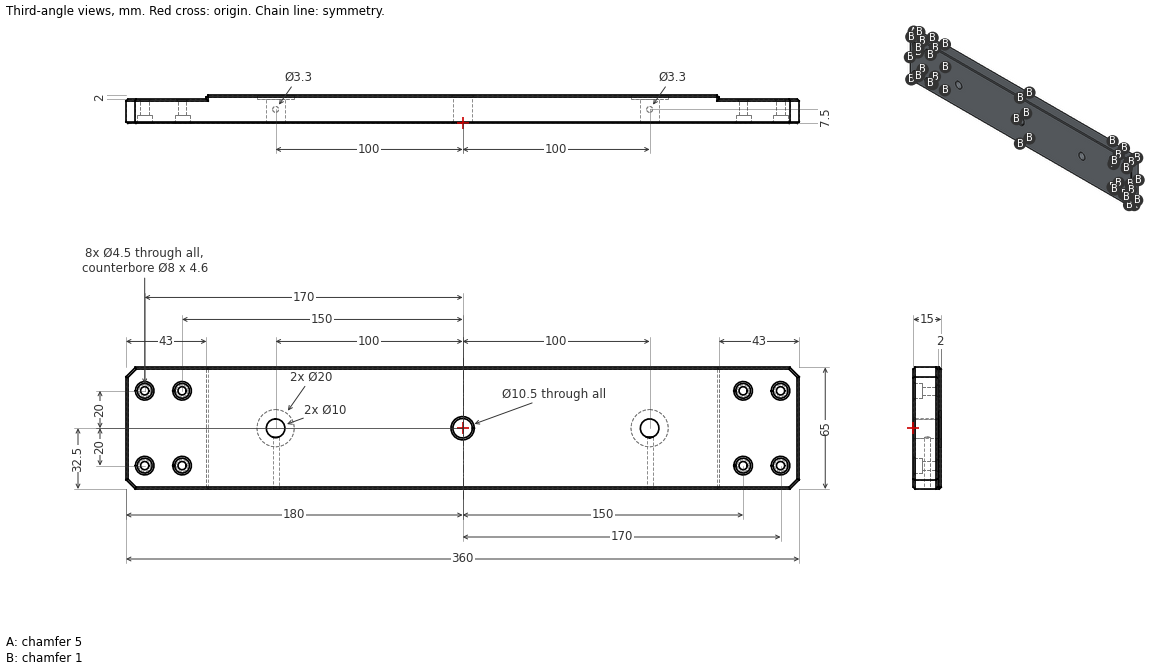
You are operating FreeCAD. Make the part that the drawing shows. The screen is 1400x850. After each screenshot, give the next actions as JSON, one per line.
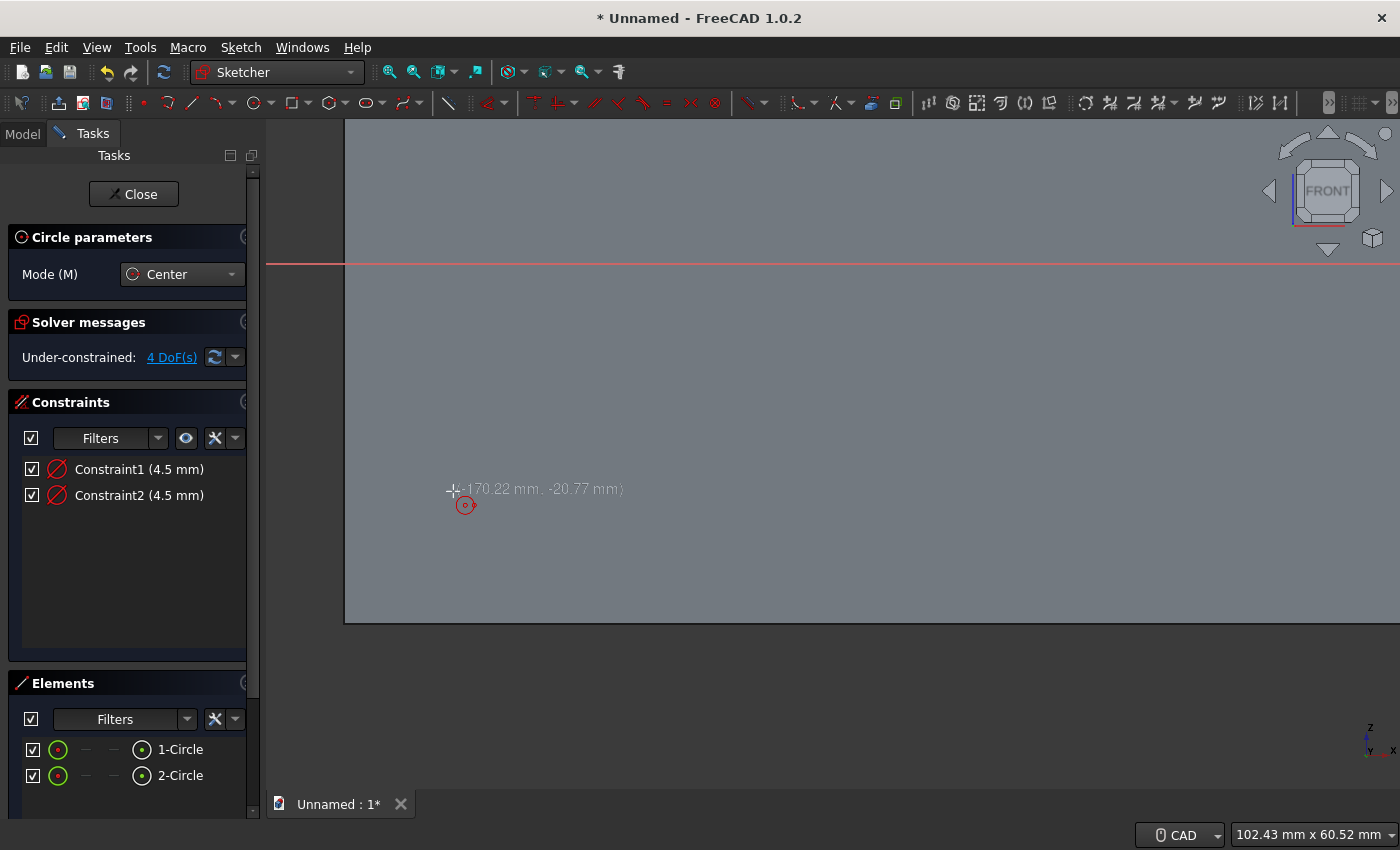
{"action": "scroll", "coordinate": [453, 492], "scroll_direction": "down", "scroll_amount": 9}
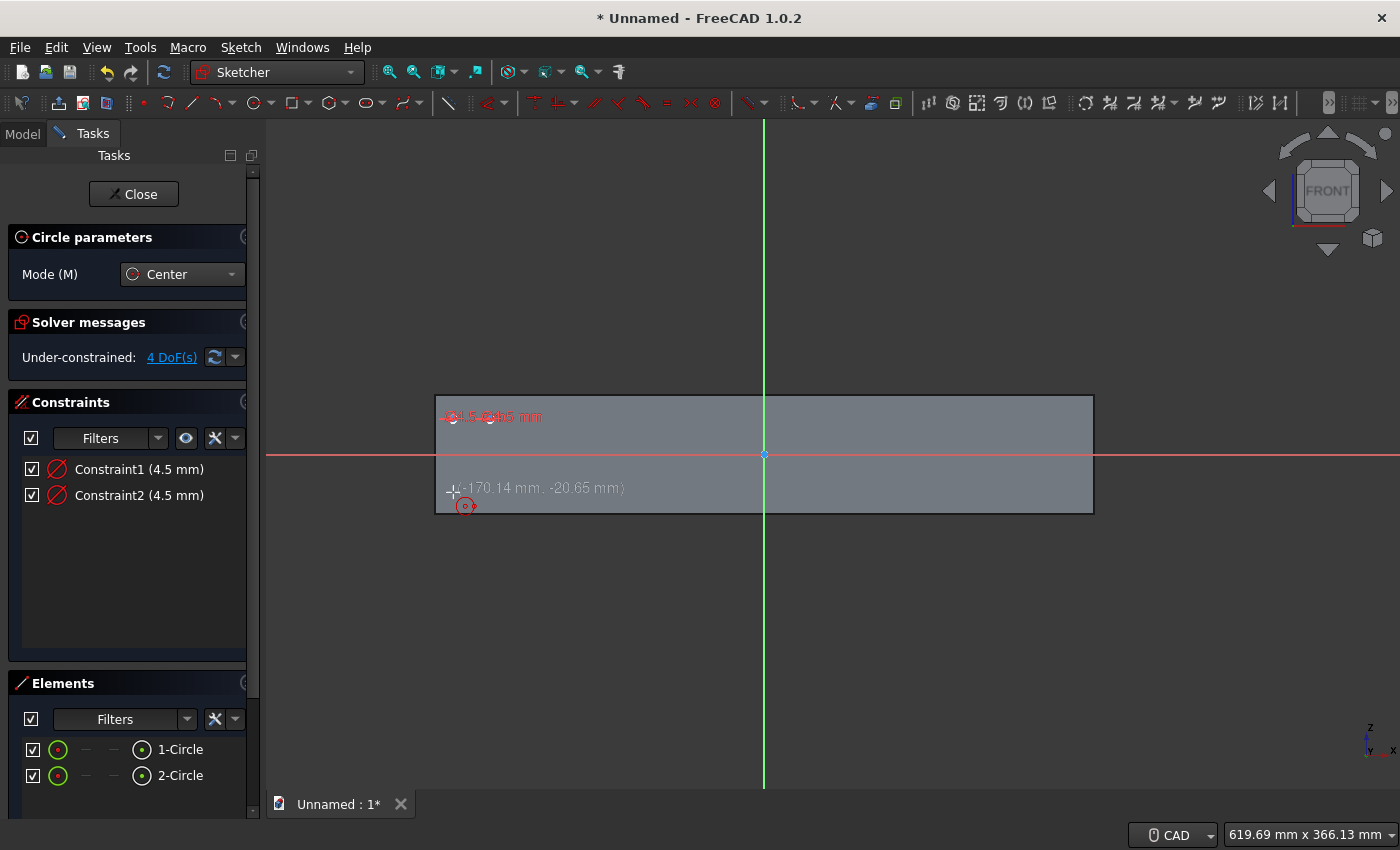
{"action": "left_click", "coordinate": [453, 491]}
{"action": "mouse_move", "coordinate": [456, 489]}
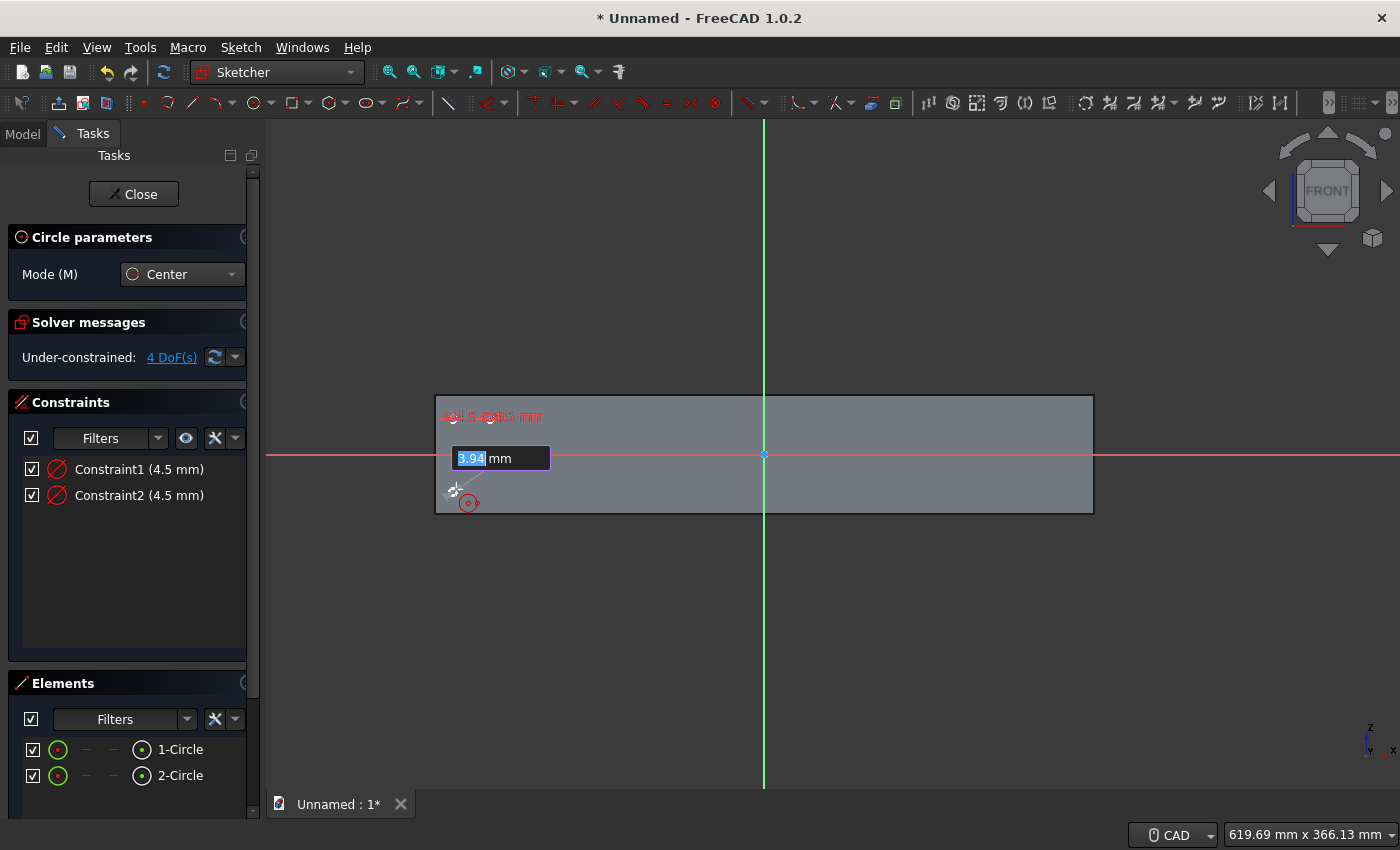
{"action": "type", "text": "4.5"}
{"action": "key", "text": "Return"}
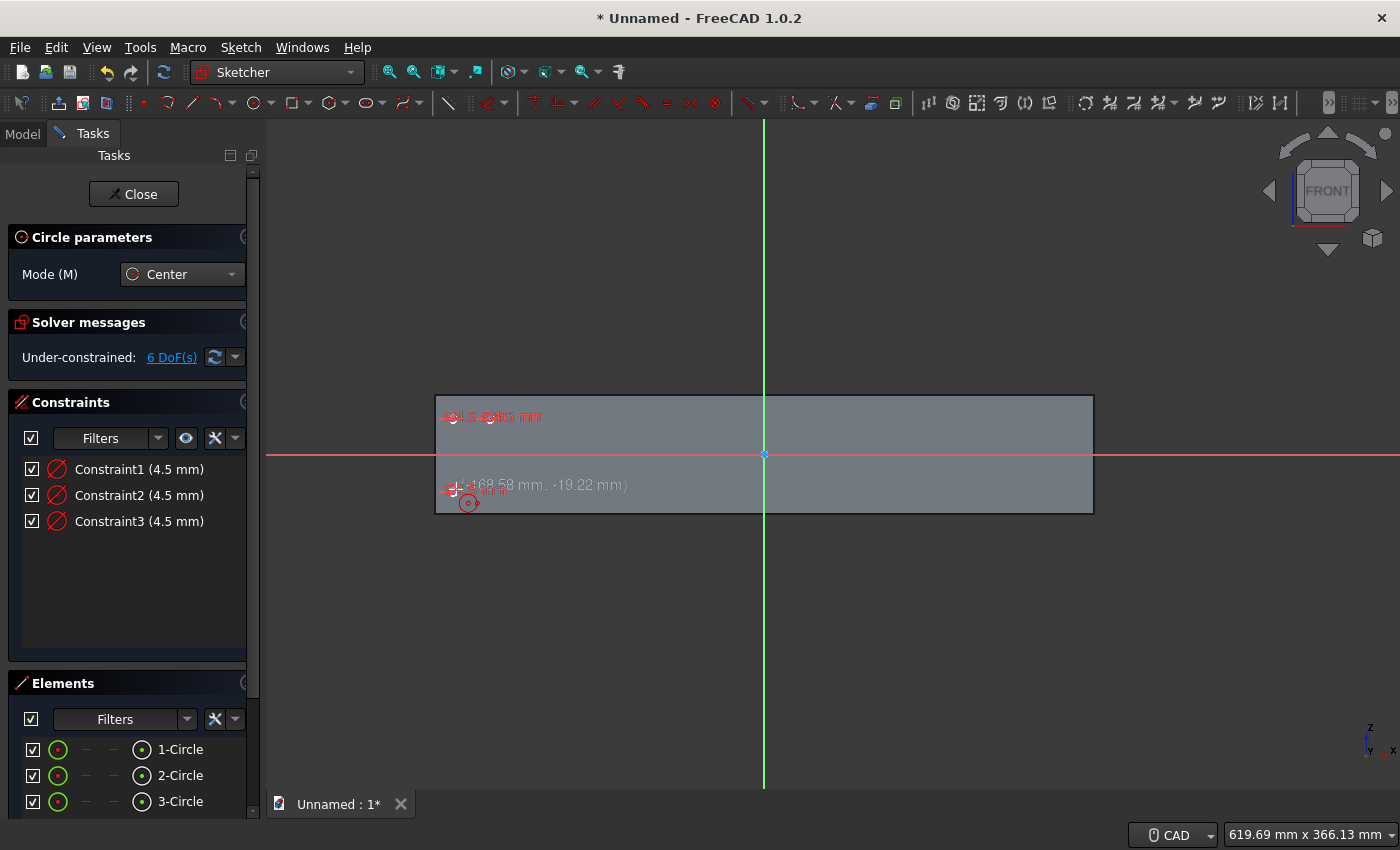
{"action": "scroll", "coordinate": [490, 491], "scroll_direction": "up", "scroll_amount": 9}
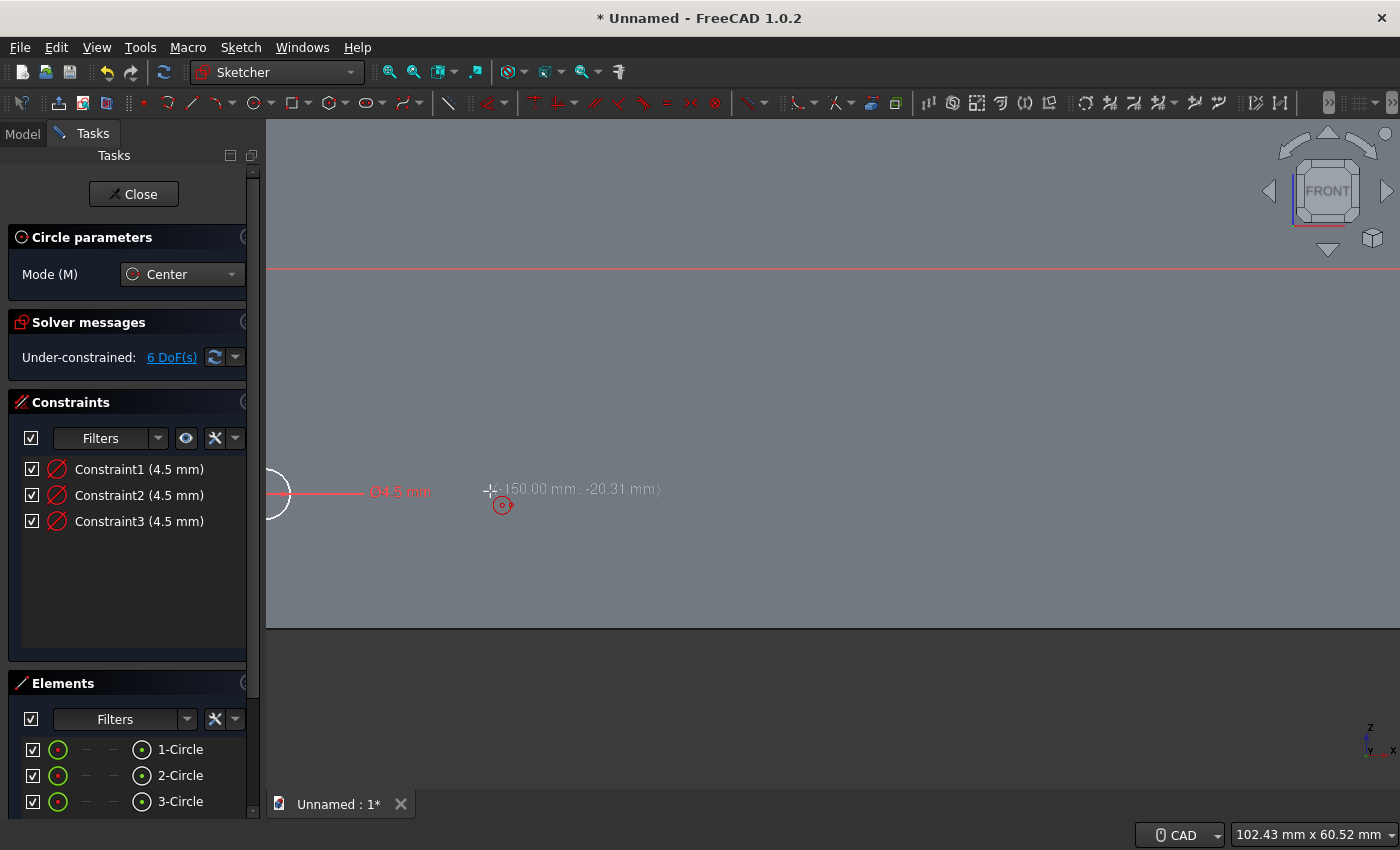
{"action": "scroll", "coordinate": [490, 491], "scroll_direction": "down", "scroll_amount": 9}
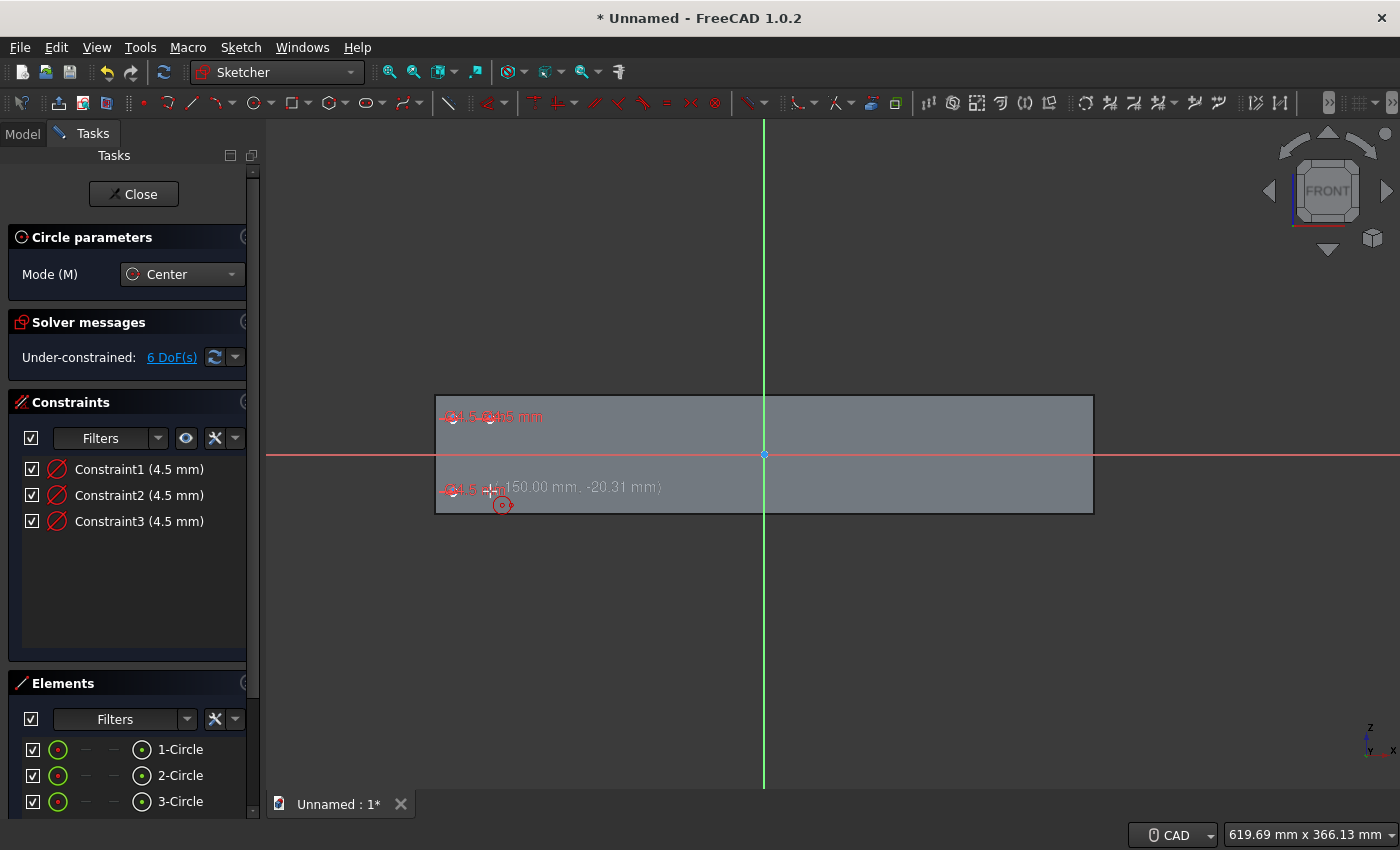
{"action": "left_click", "coordinate": [490, 491]}
{"action": "mouse_move", "coordinate": [493, 489]}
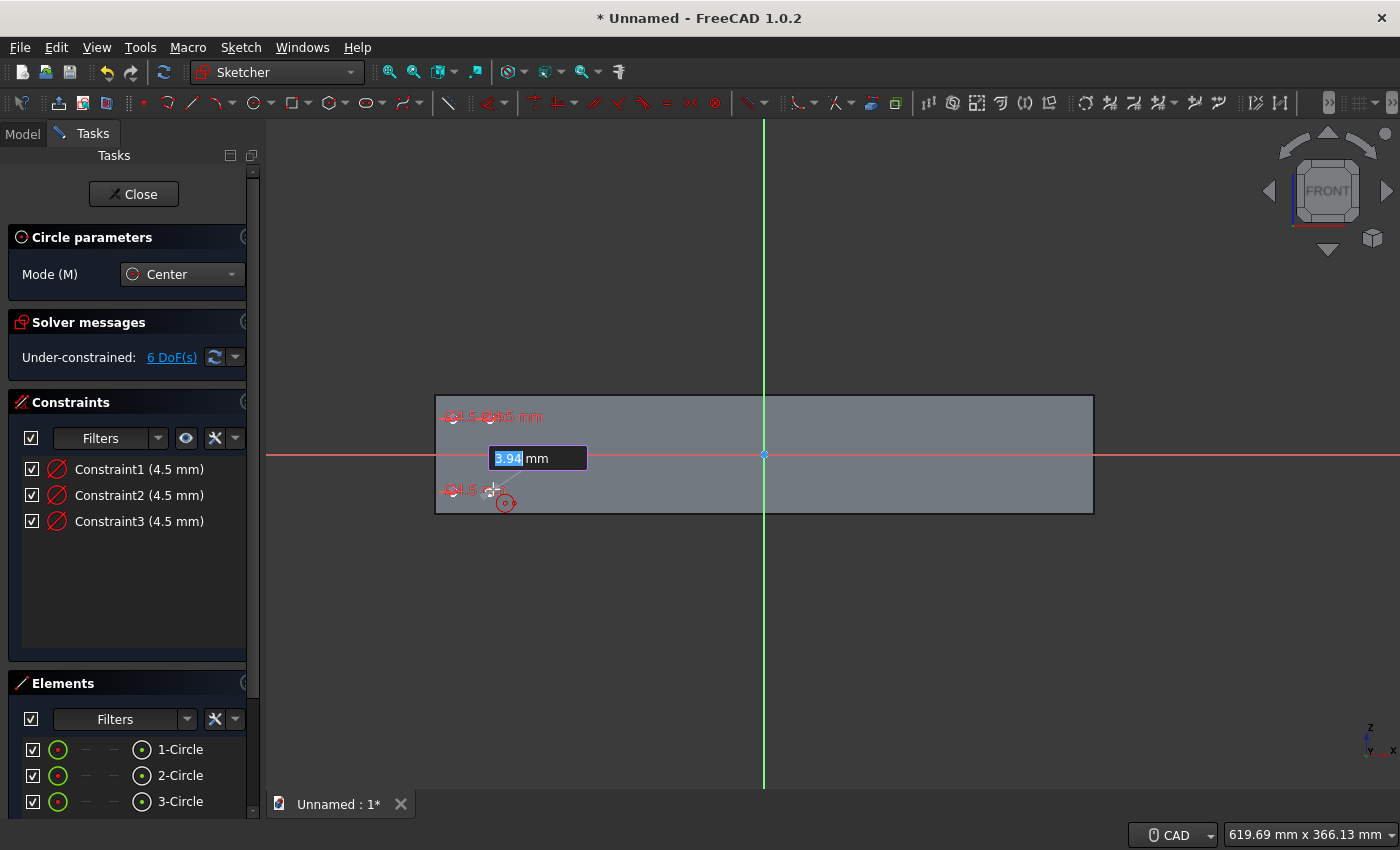
{"action": "type", "text": "4.5"}
{"action": "key", "text": "Return"}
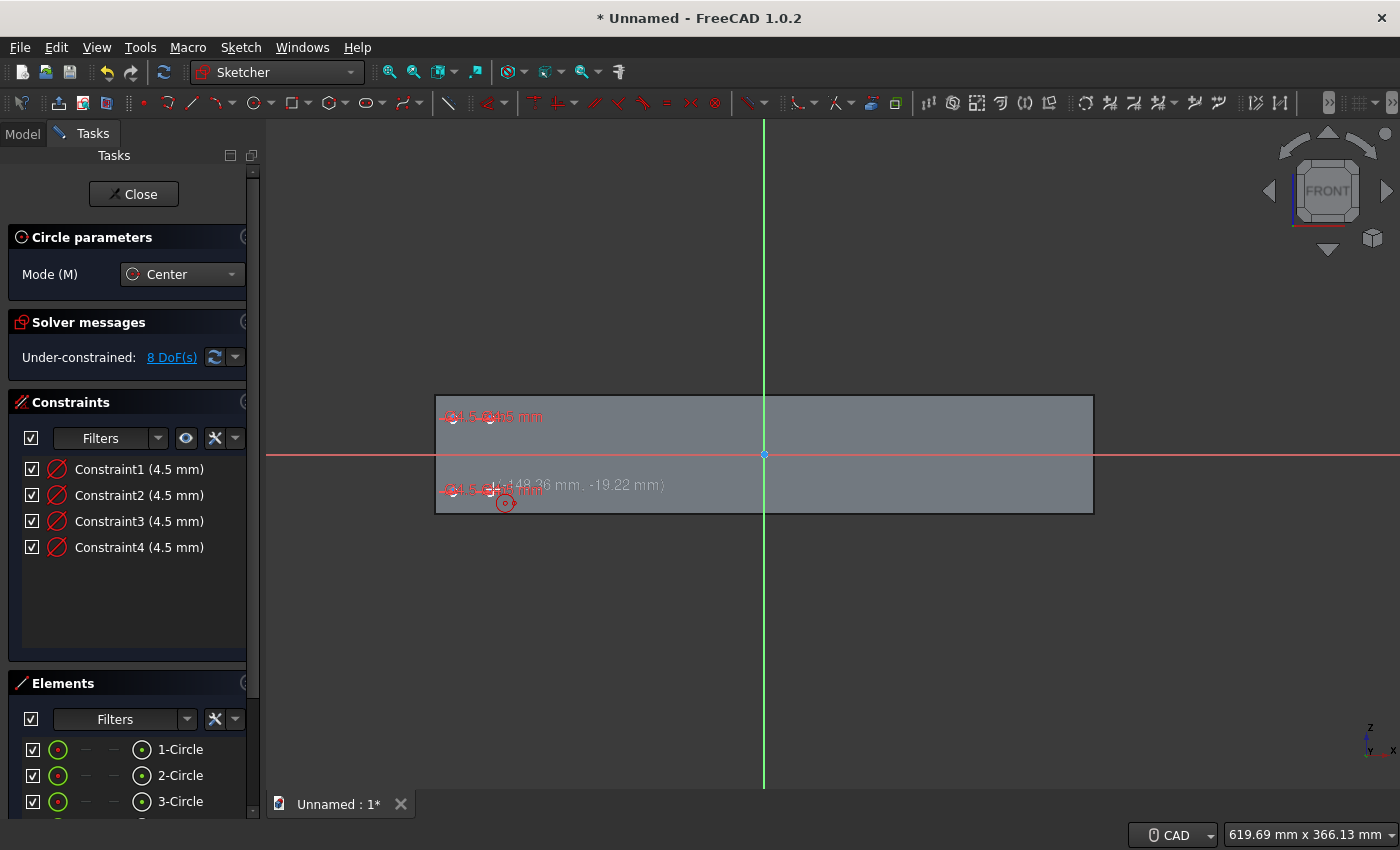
{"action": "scroll", "coordinate": [1039, 491], "scroll_direction": "up", "scroll_amount": 9}